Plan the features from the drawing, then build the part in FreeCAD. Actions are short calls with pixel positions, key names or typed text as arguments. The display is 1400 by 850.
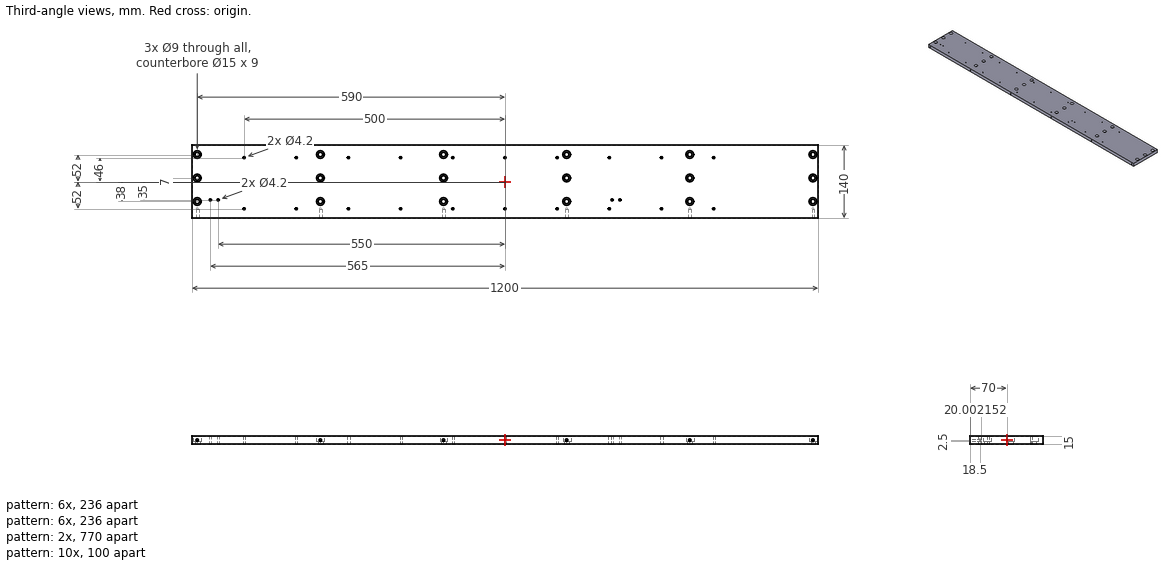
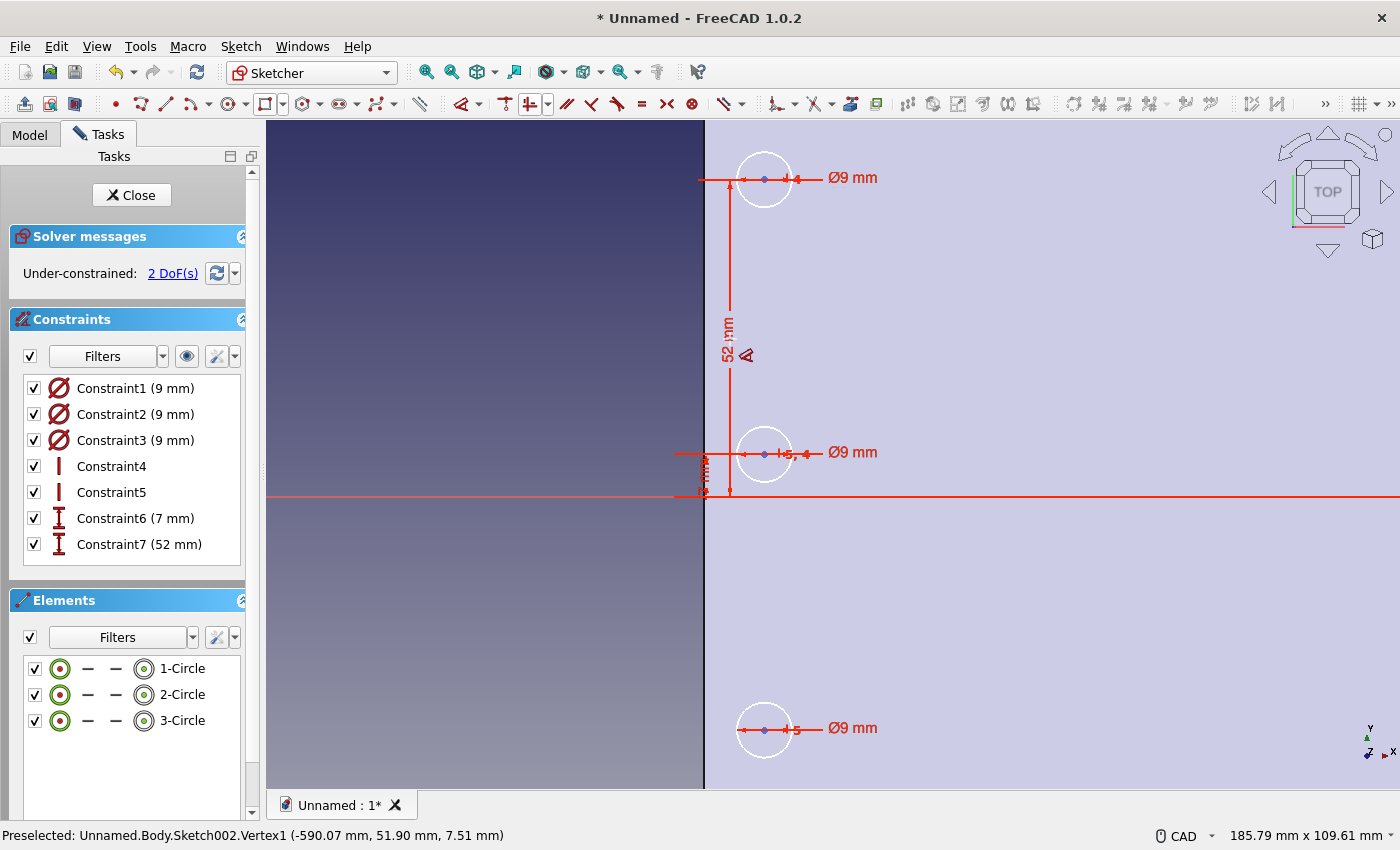
click(764, 730)
click(730, 614)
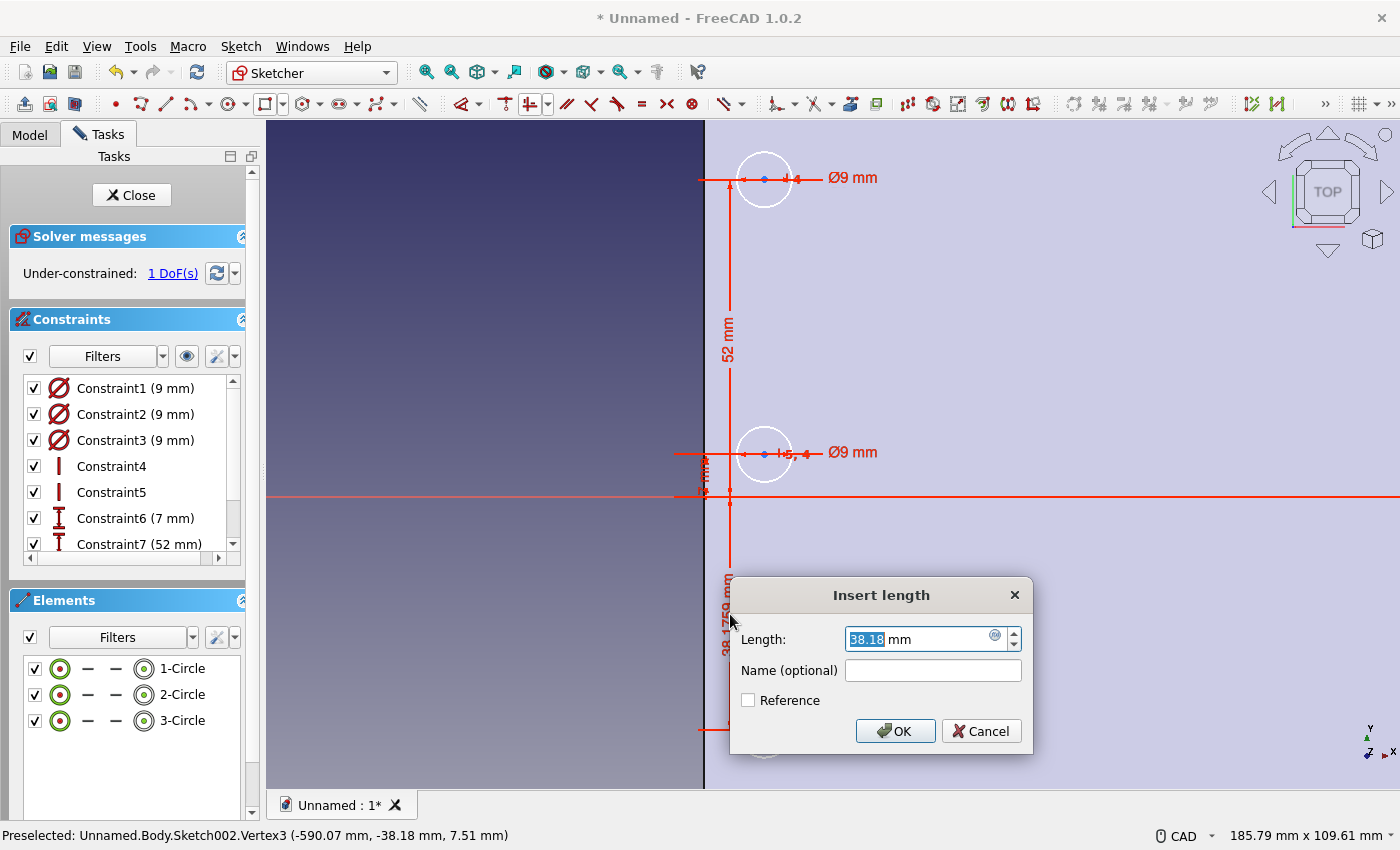
text(38)
key(Return)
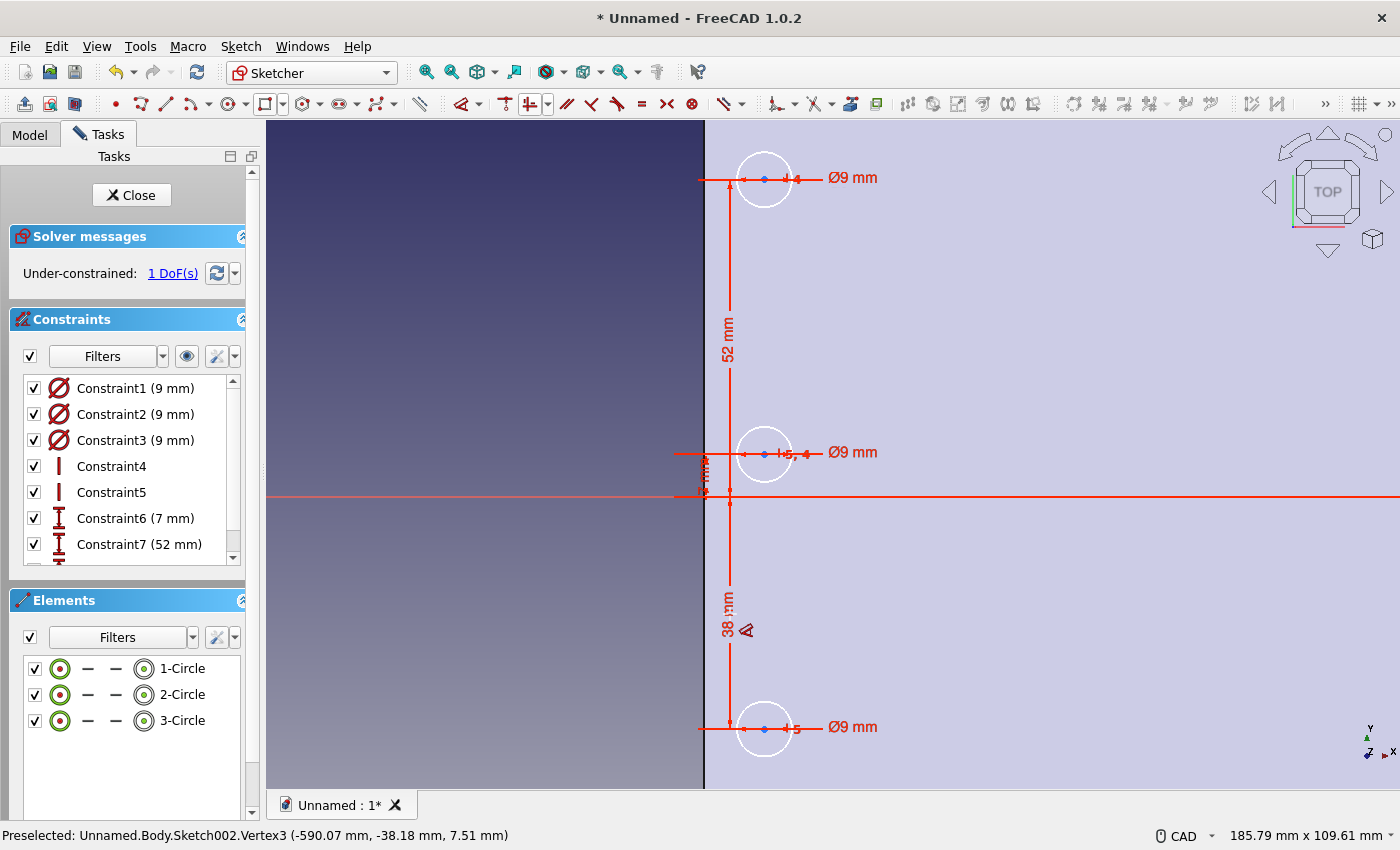
click(764, 180)
click(1000, 531)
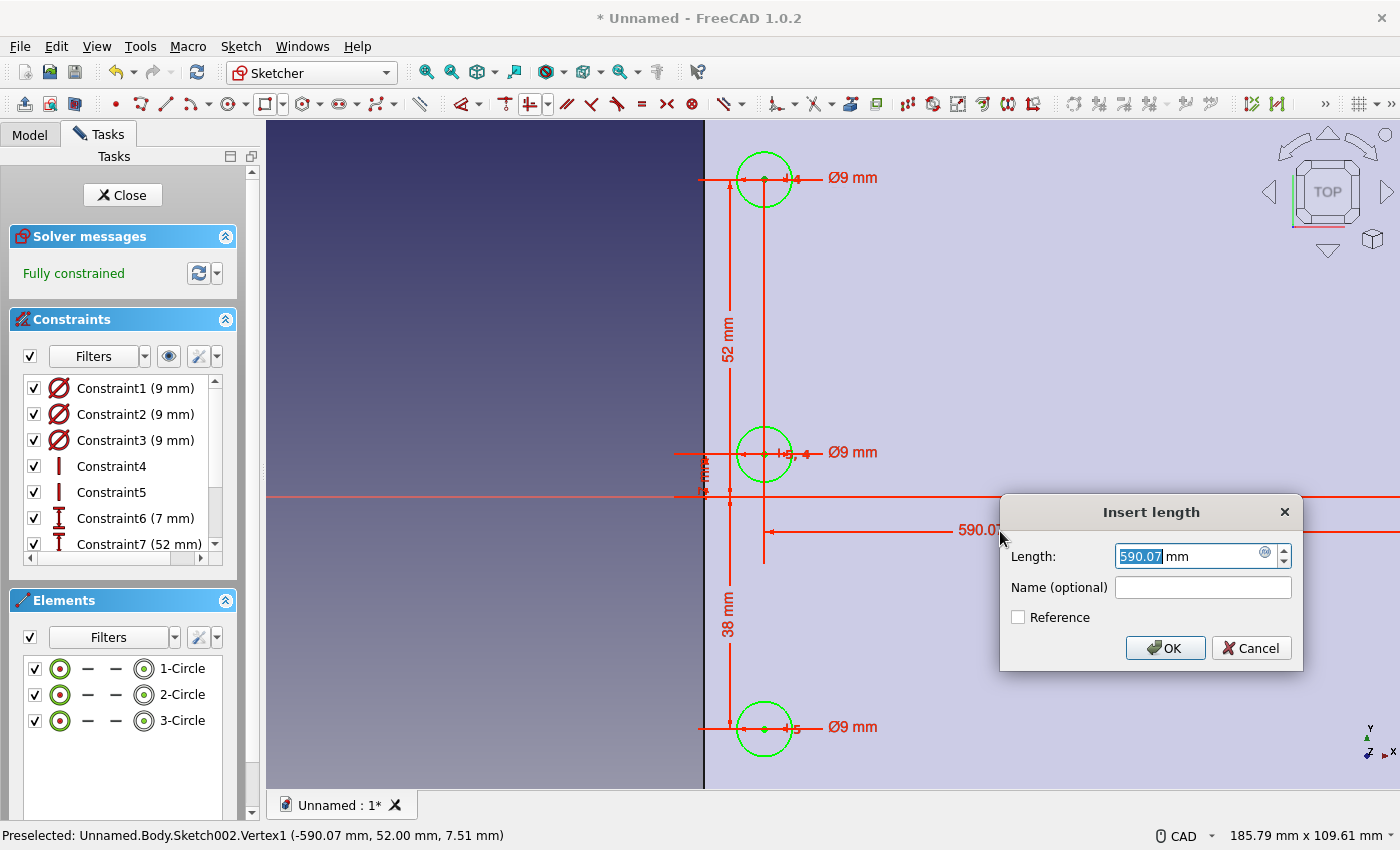
text(590)
key(Return)
key(Escape)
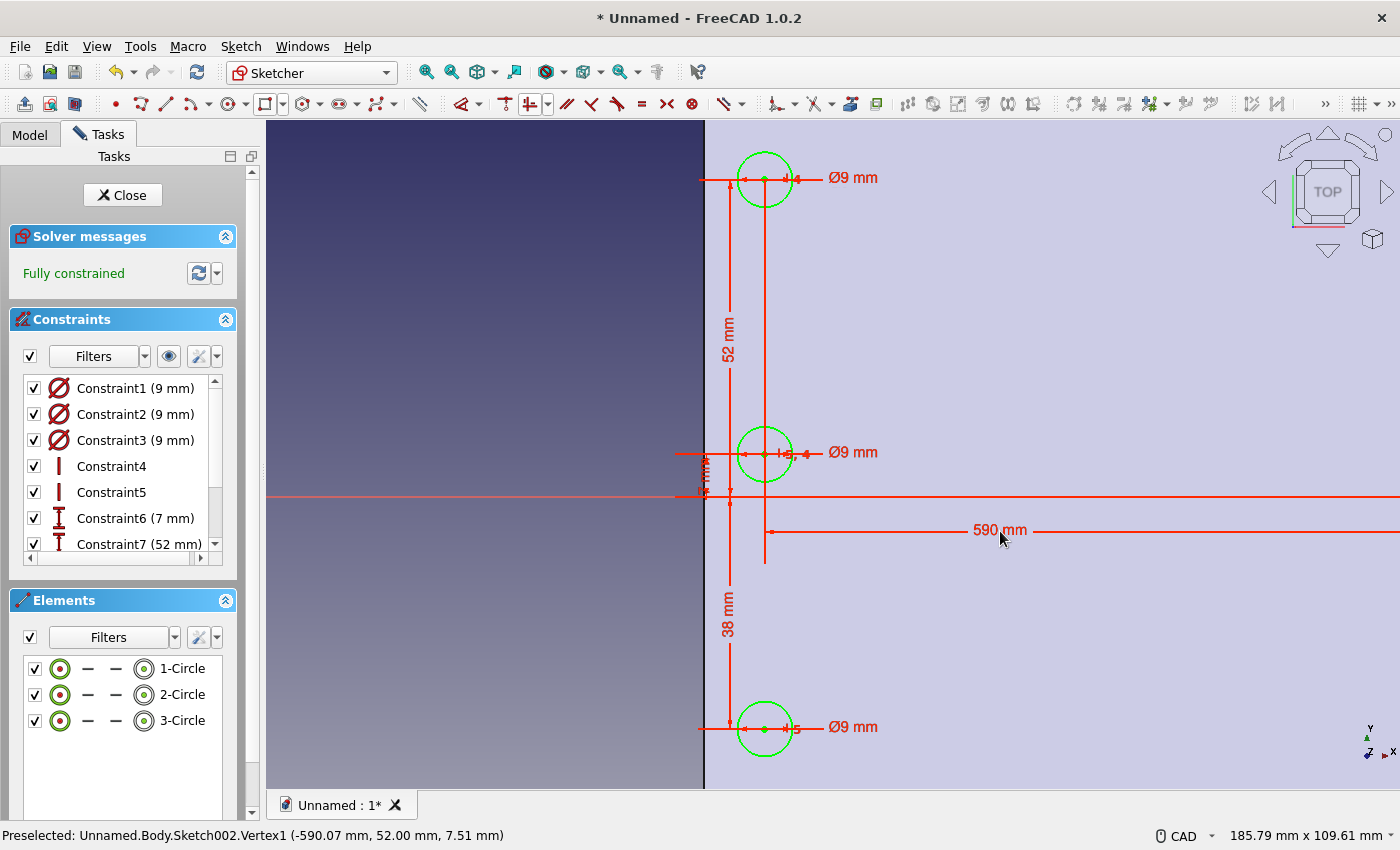
click(123, 195)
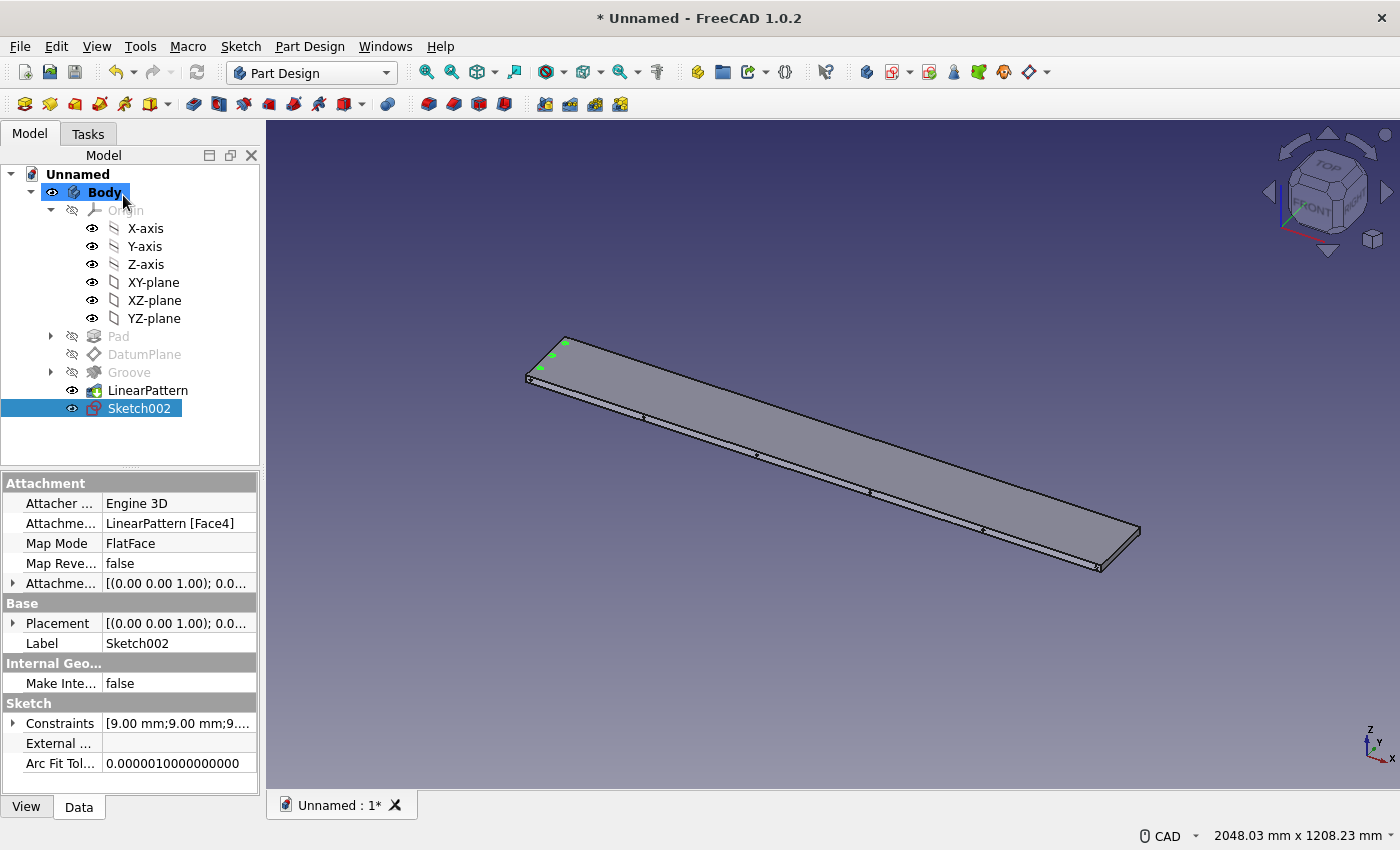
click(219, 104)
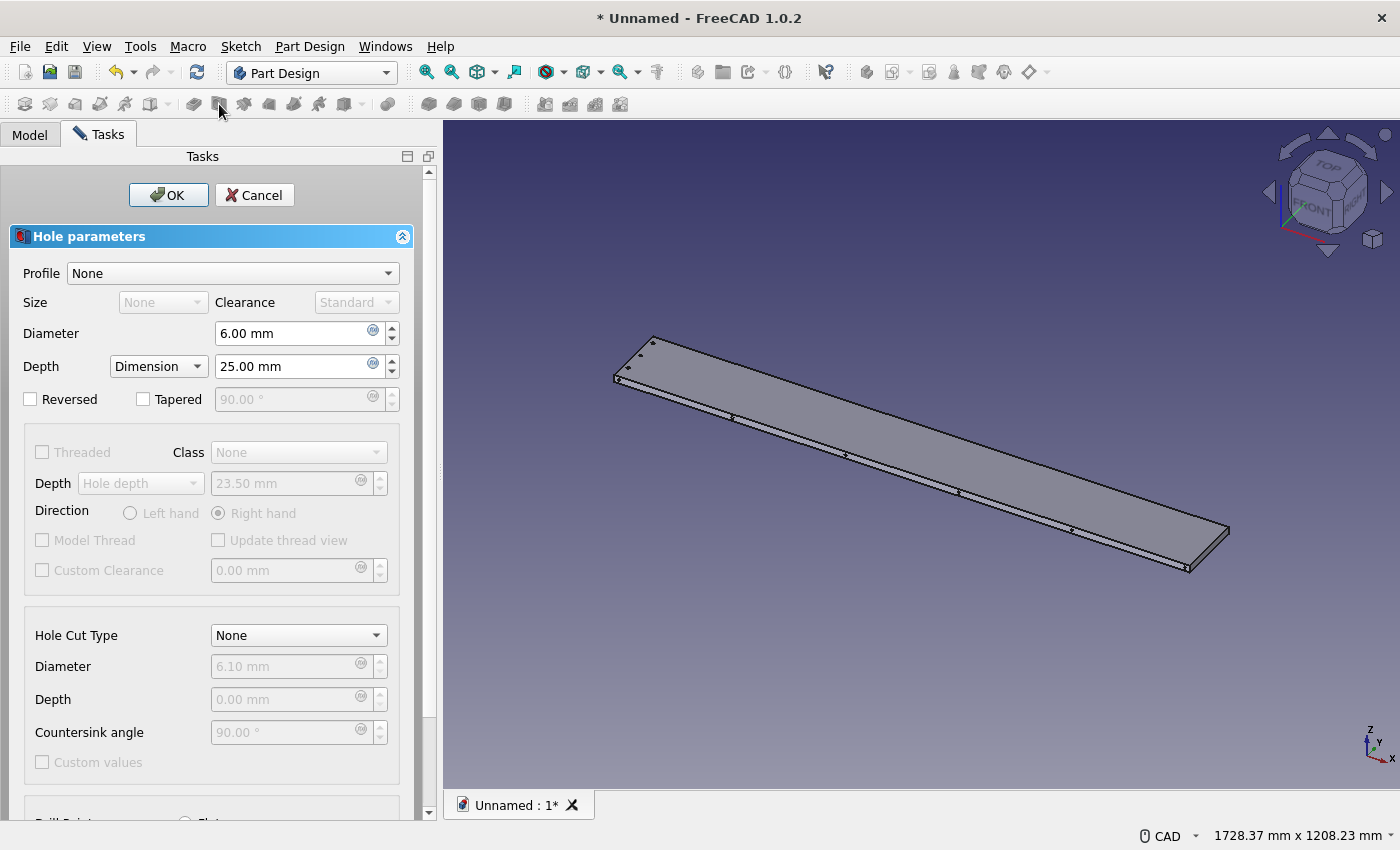
triple_click(300, 334)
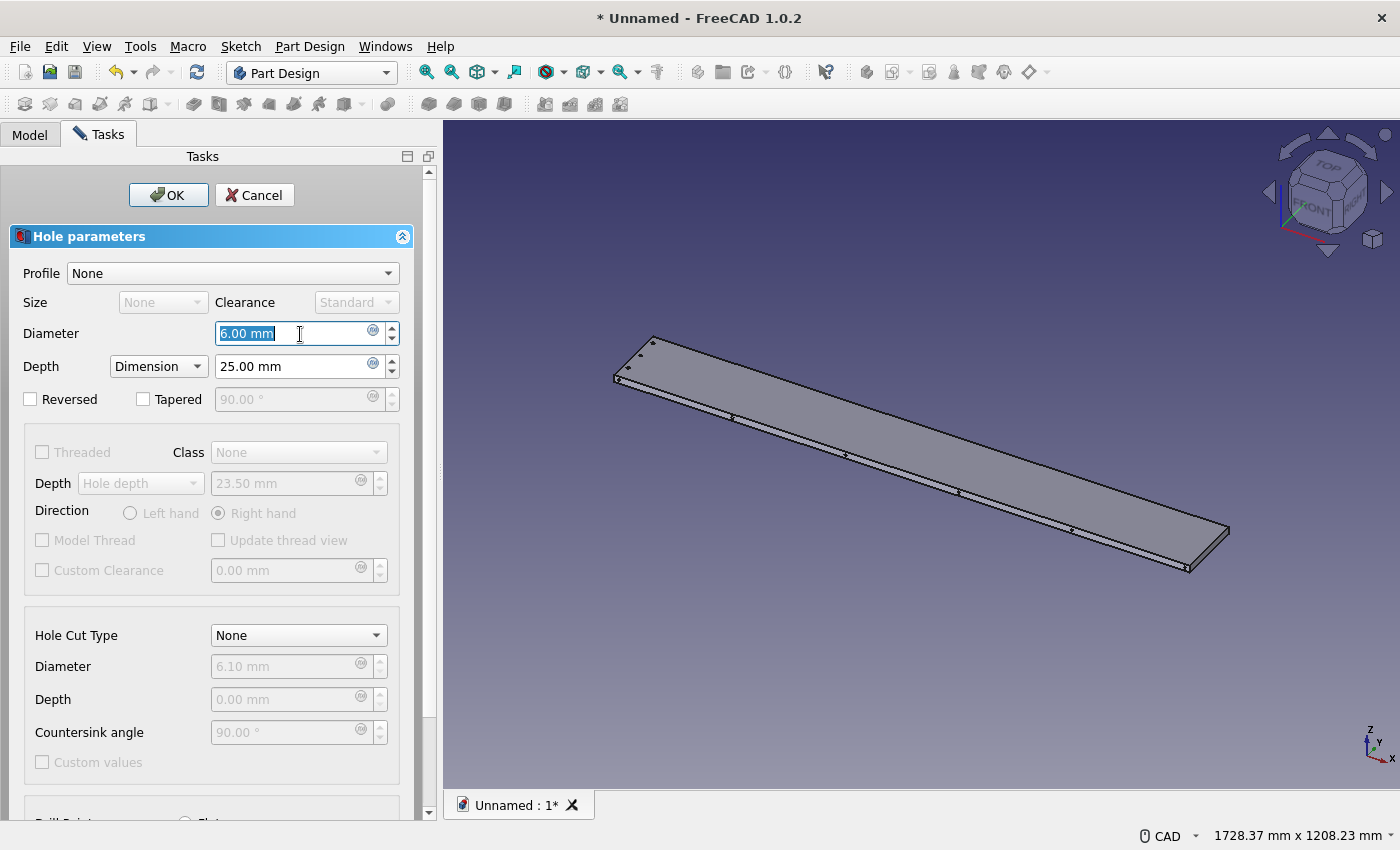
text(9)
key(Tab)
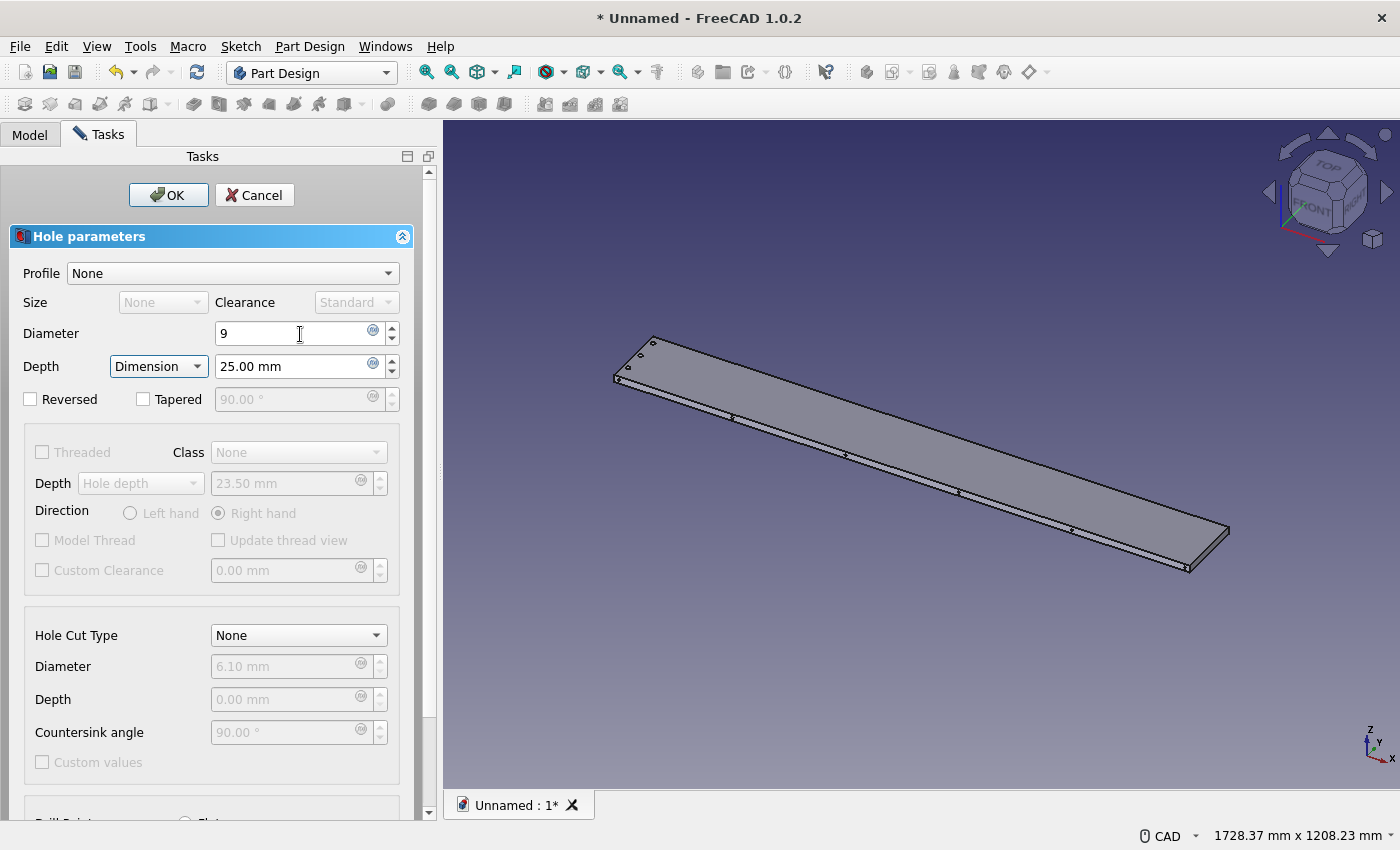
click(160, 366)